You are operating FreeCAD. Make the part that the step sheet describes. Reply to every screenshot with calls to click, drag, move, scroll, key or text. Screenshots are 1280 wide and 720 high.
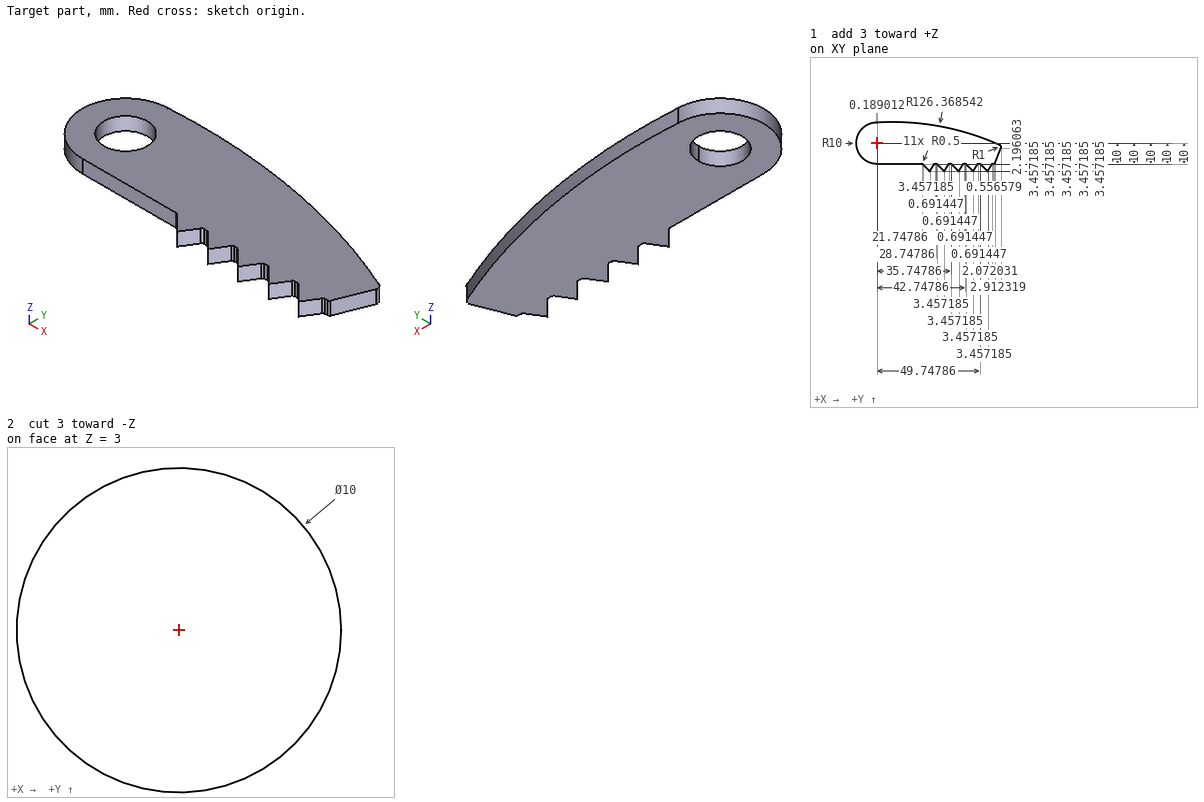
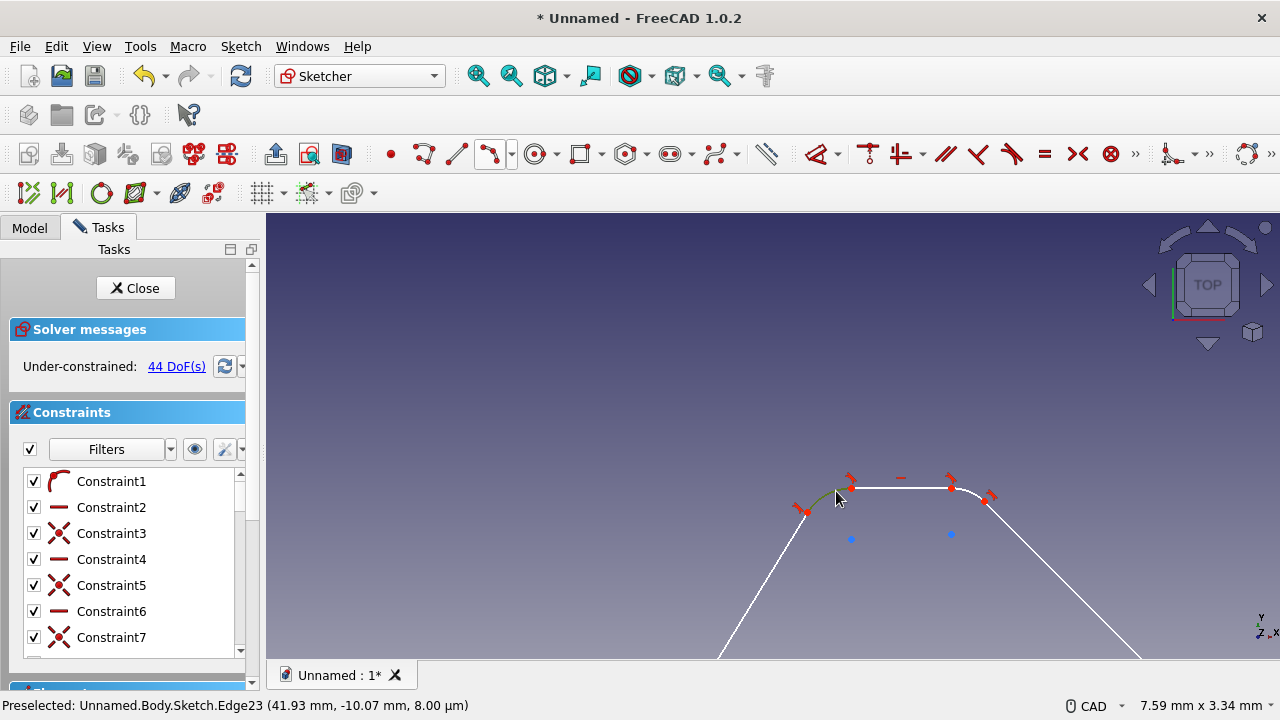
click(976, 495)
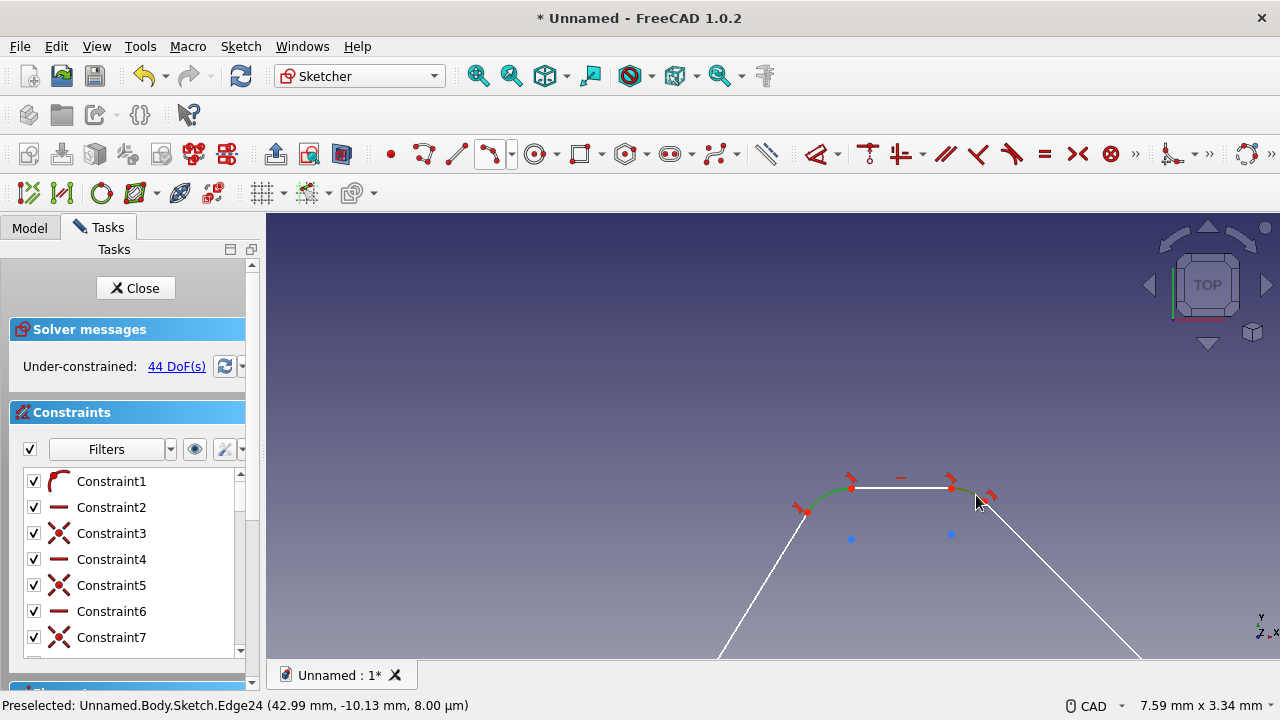
scroll(842, 504, down, 14)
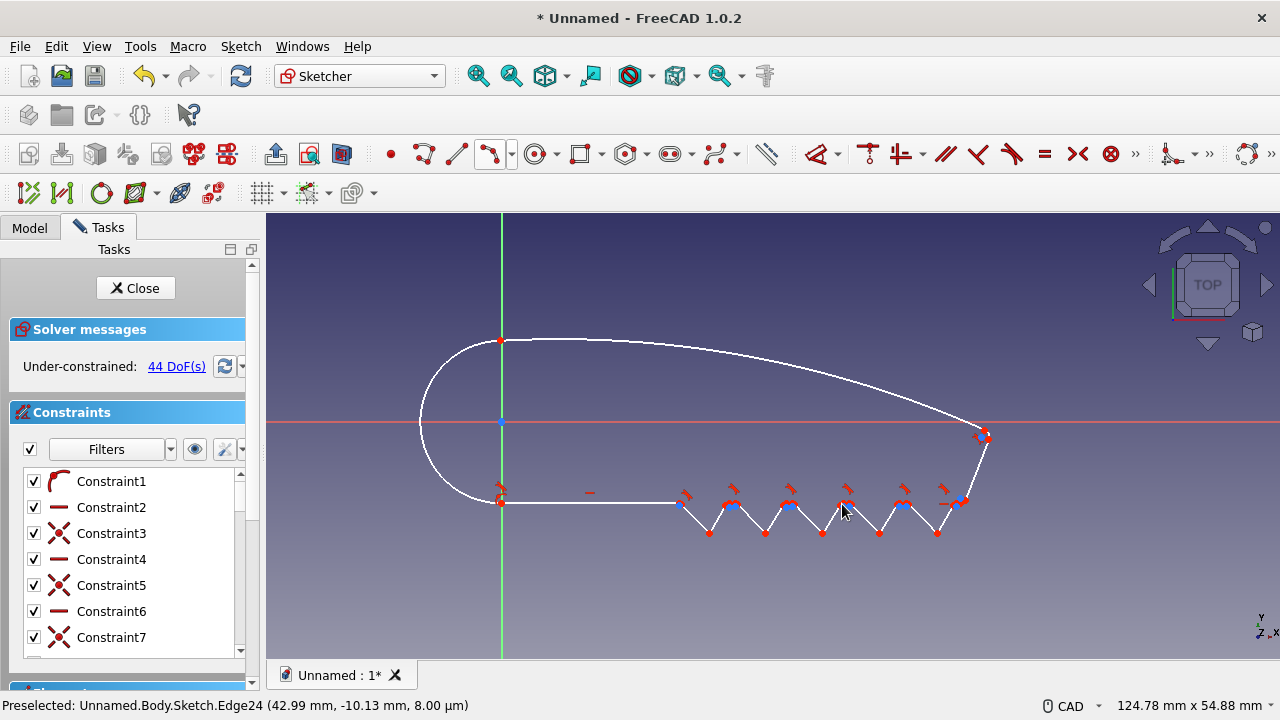
scroll(899, 503, up, 14)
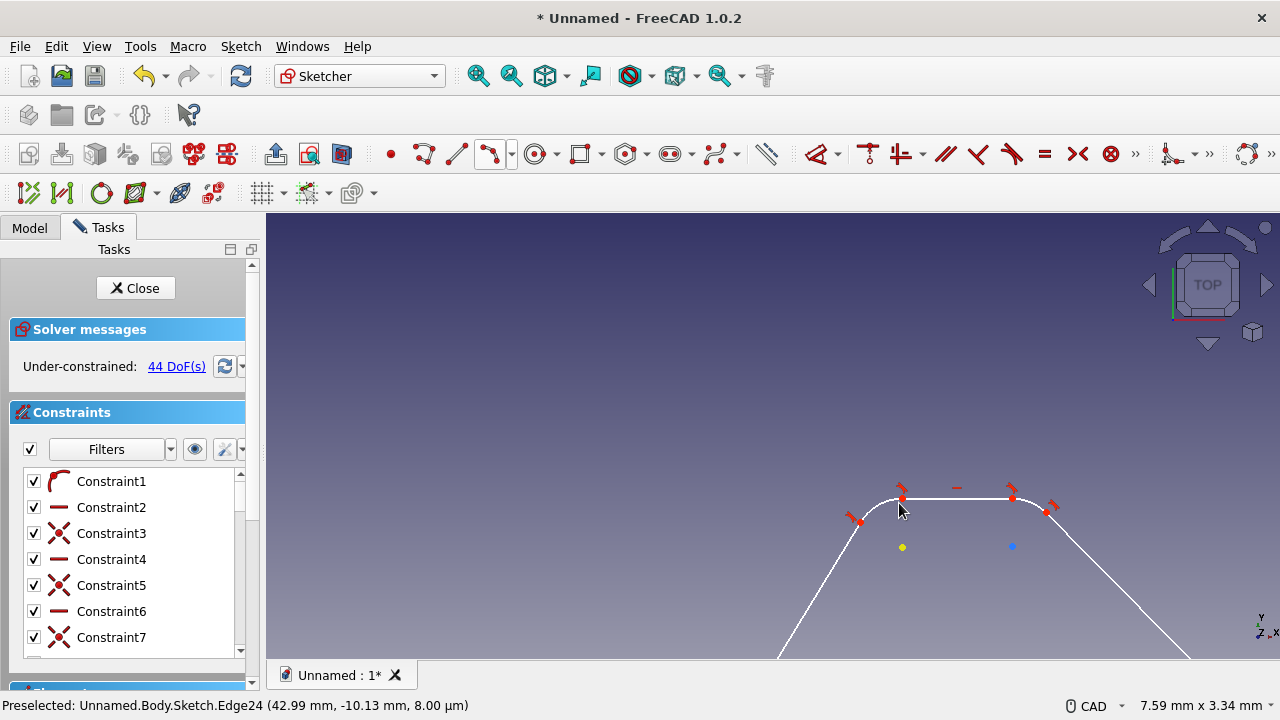
click(888, 501)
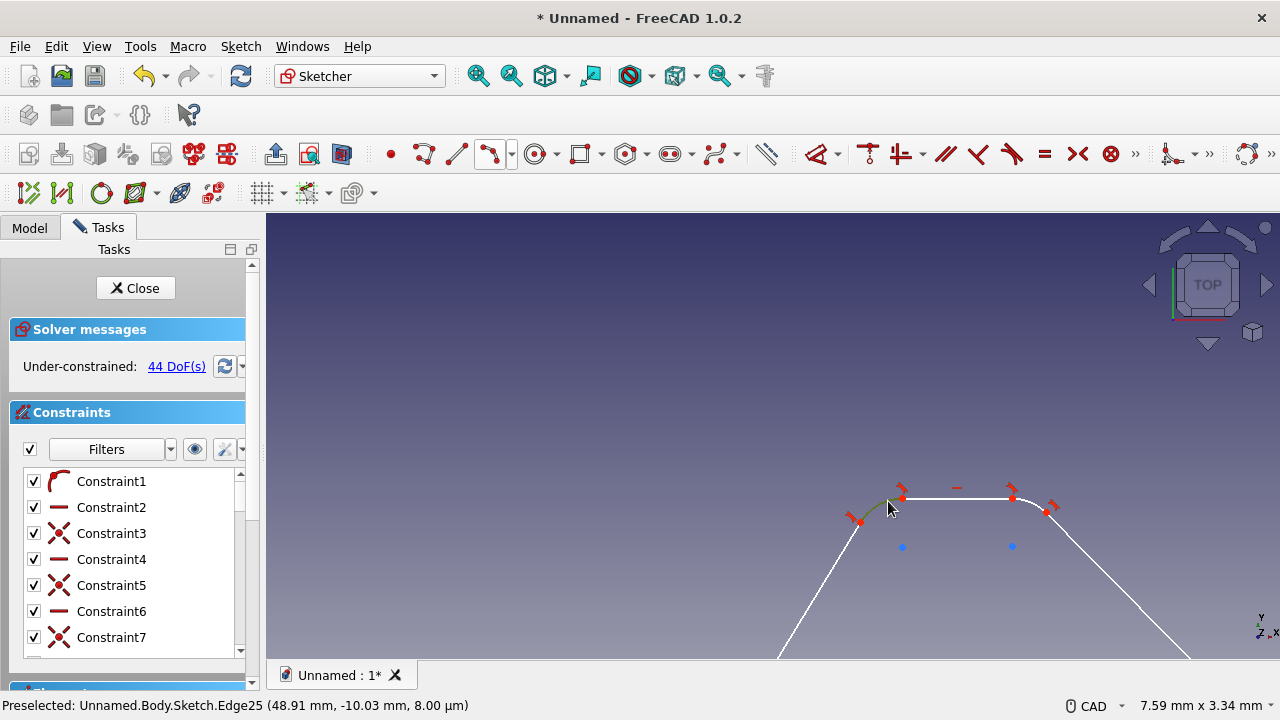
click(1037, 506)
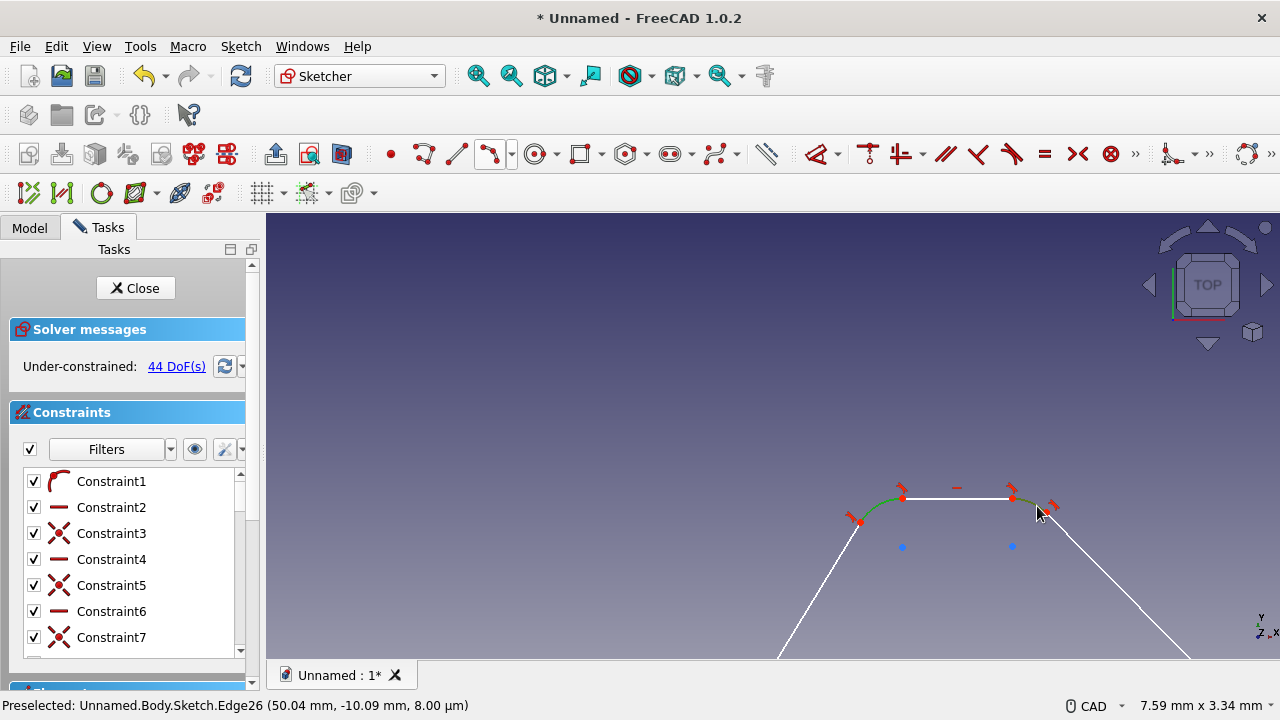
scroll(899, 503, down, 14)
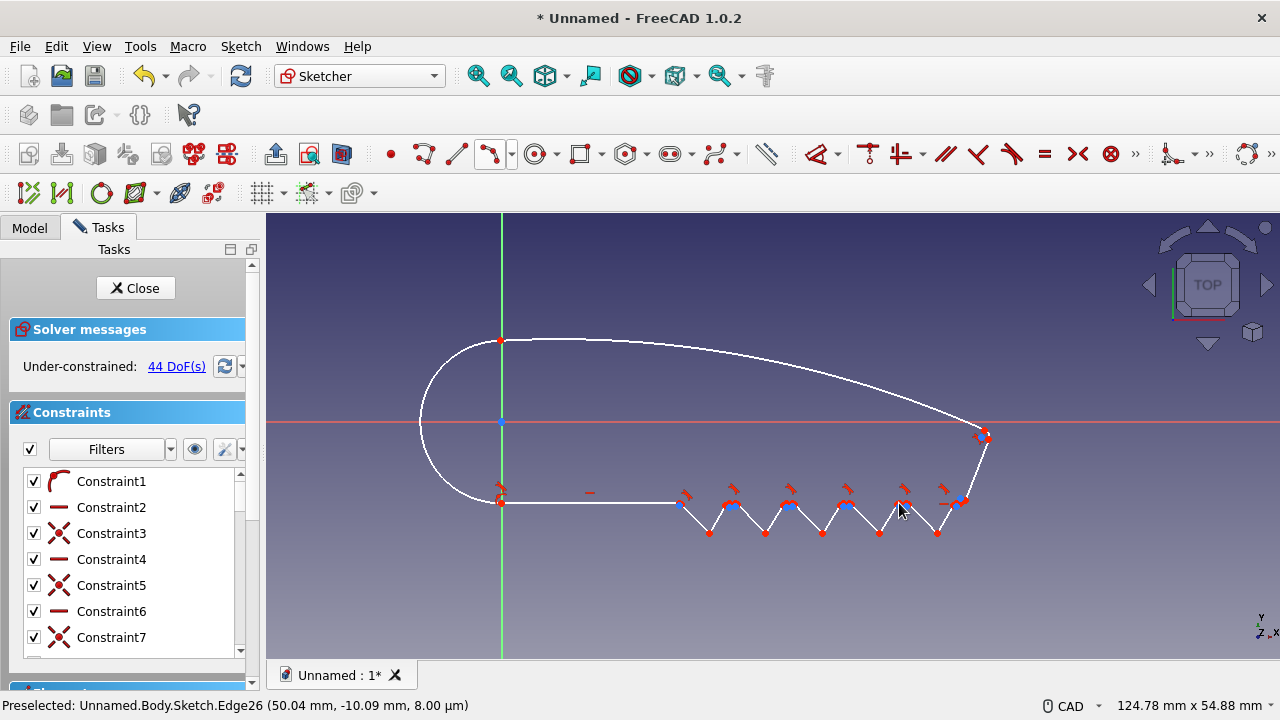
scroll(956, 504, up, 13)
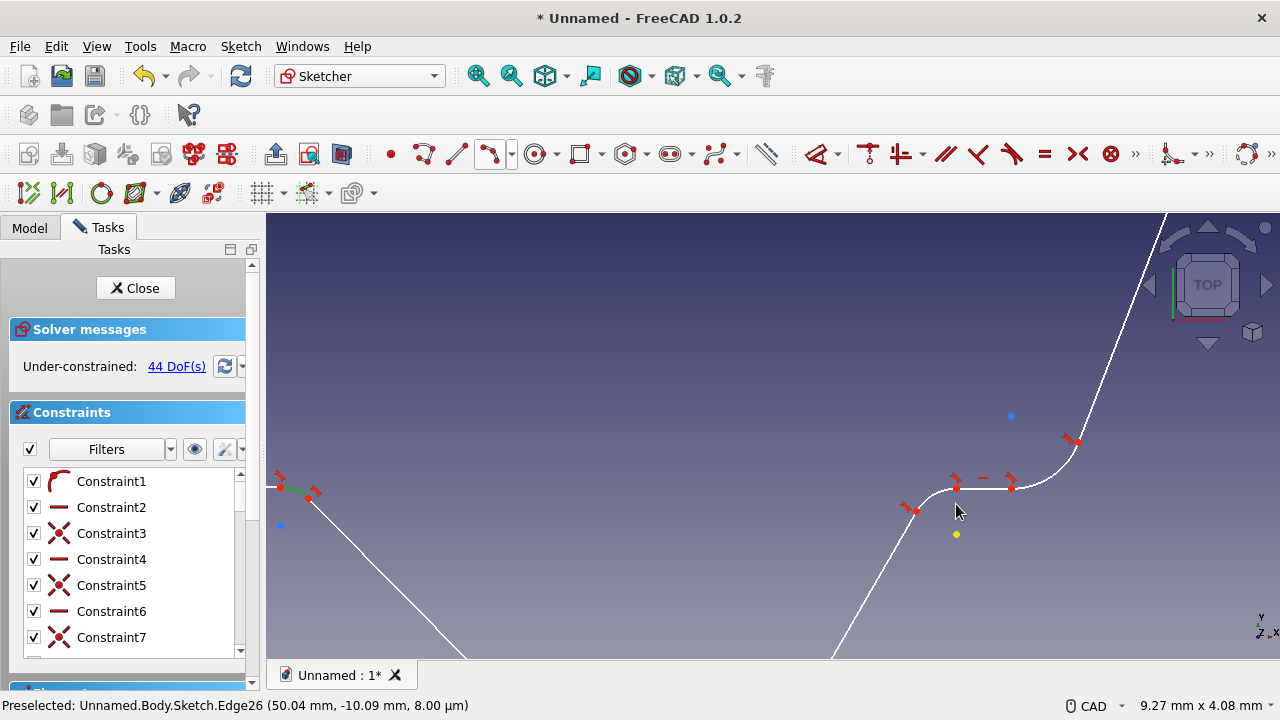
click(942, 491)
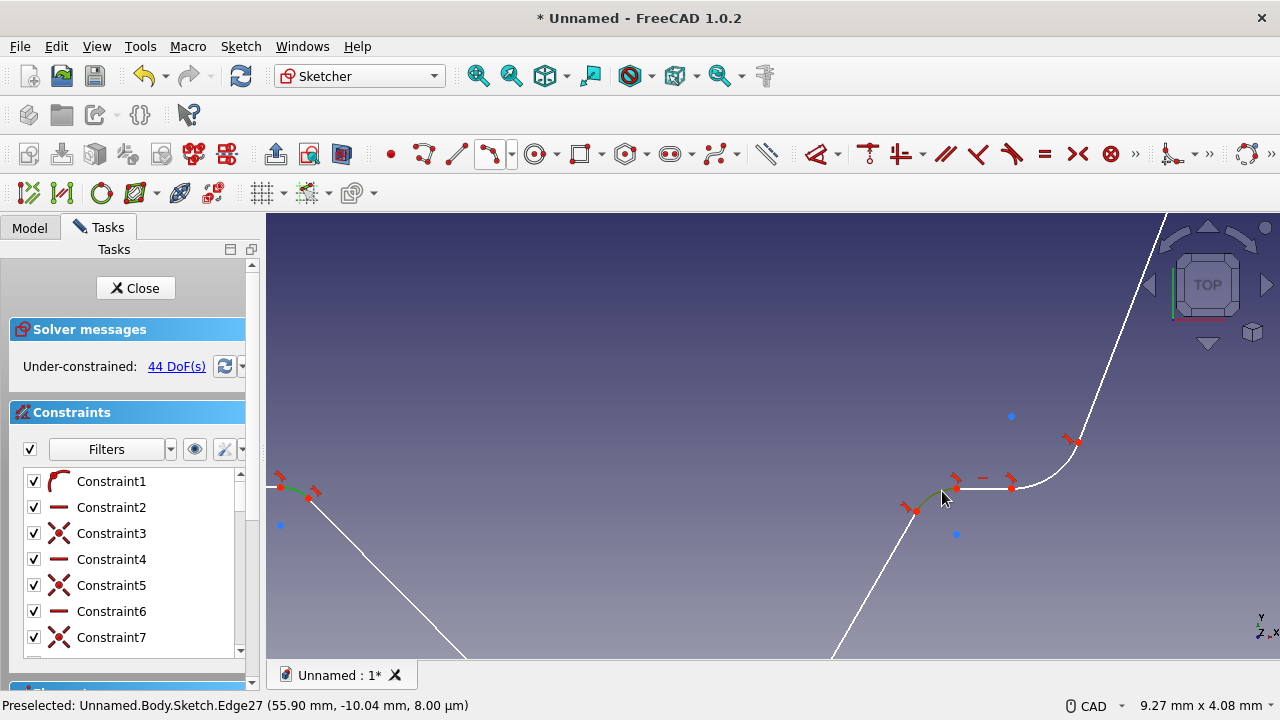
click(1037, 484)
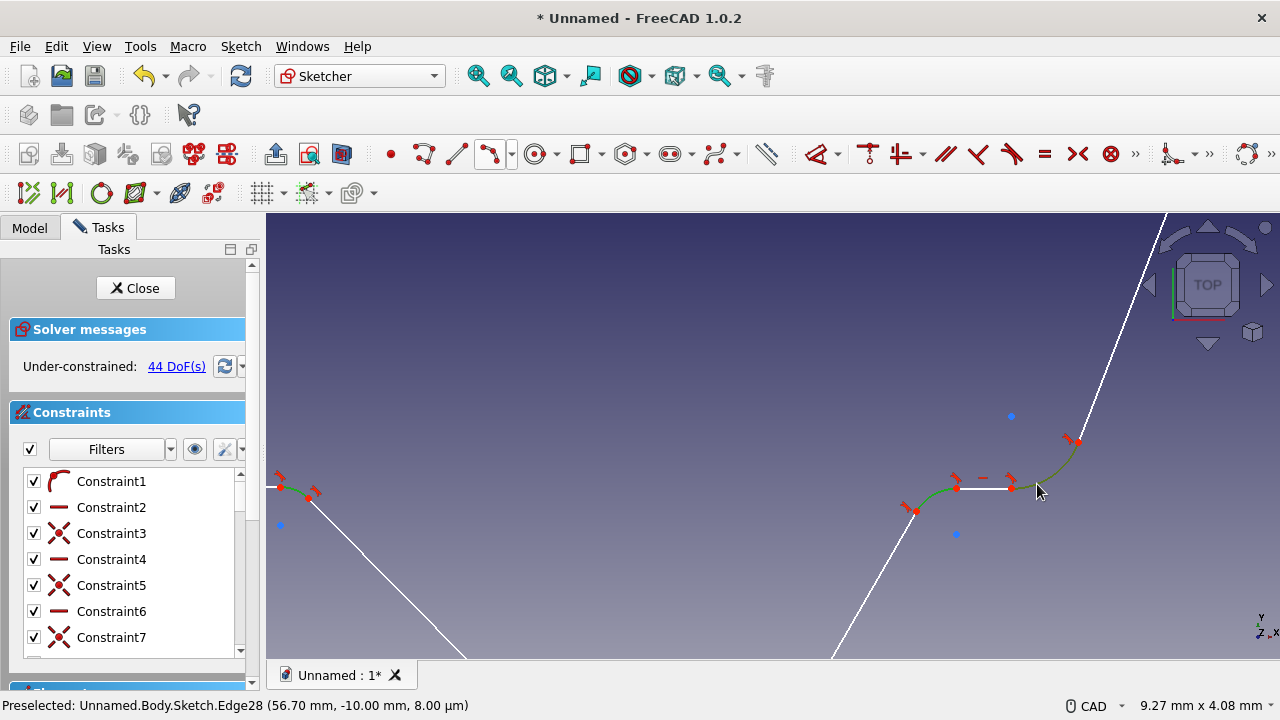
click(1045, 154)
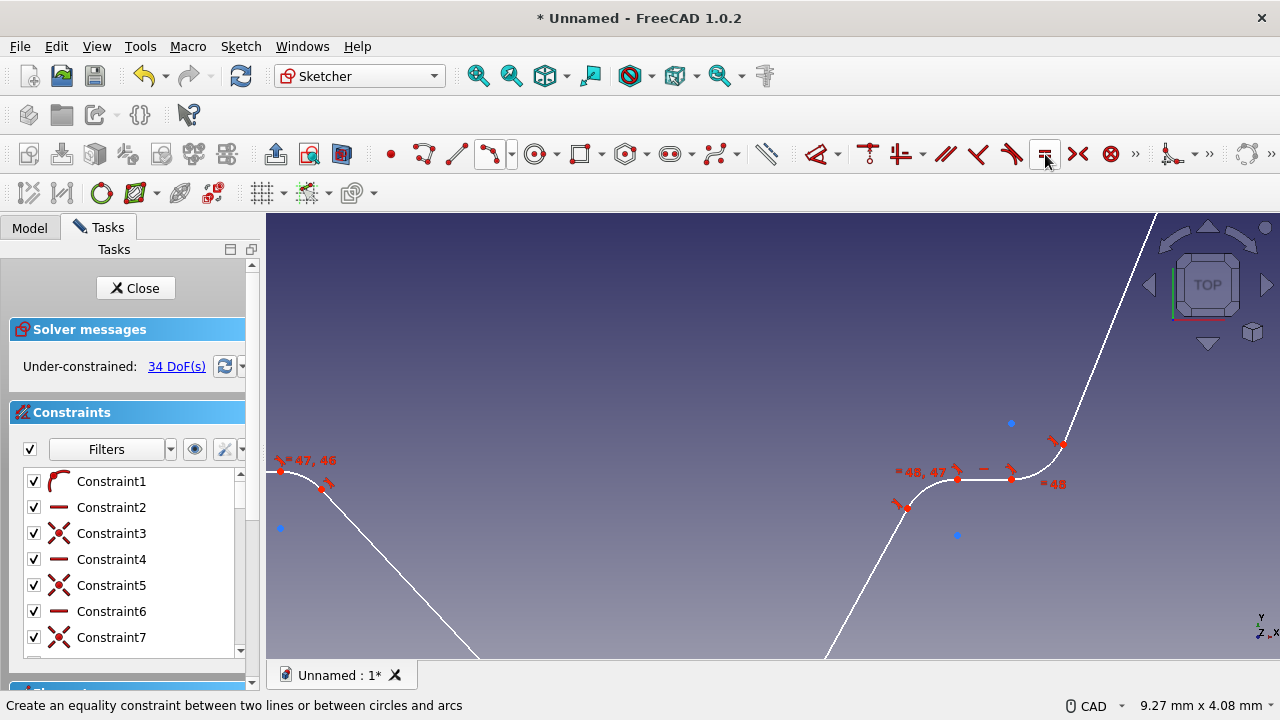
scroll(956, 504, down, 13)